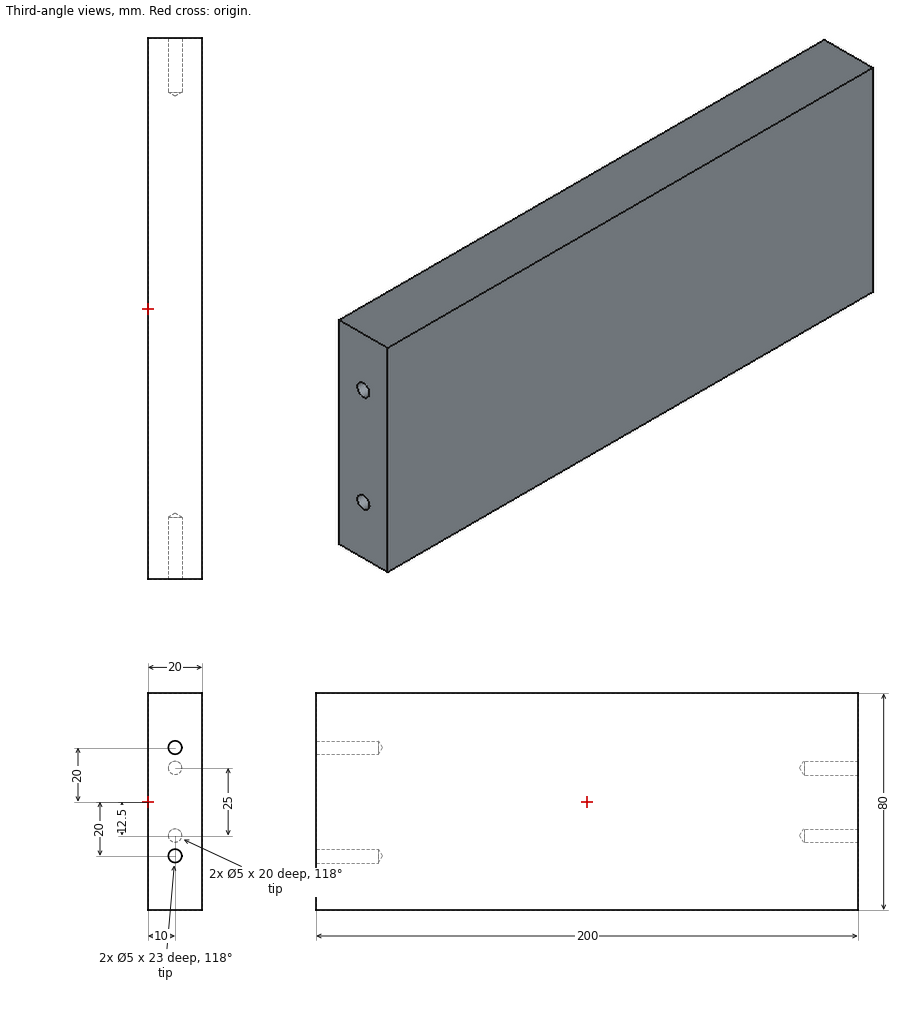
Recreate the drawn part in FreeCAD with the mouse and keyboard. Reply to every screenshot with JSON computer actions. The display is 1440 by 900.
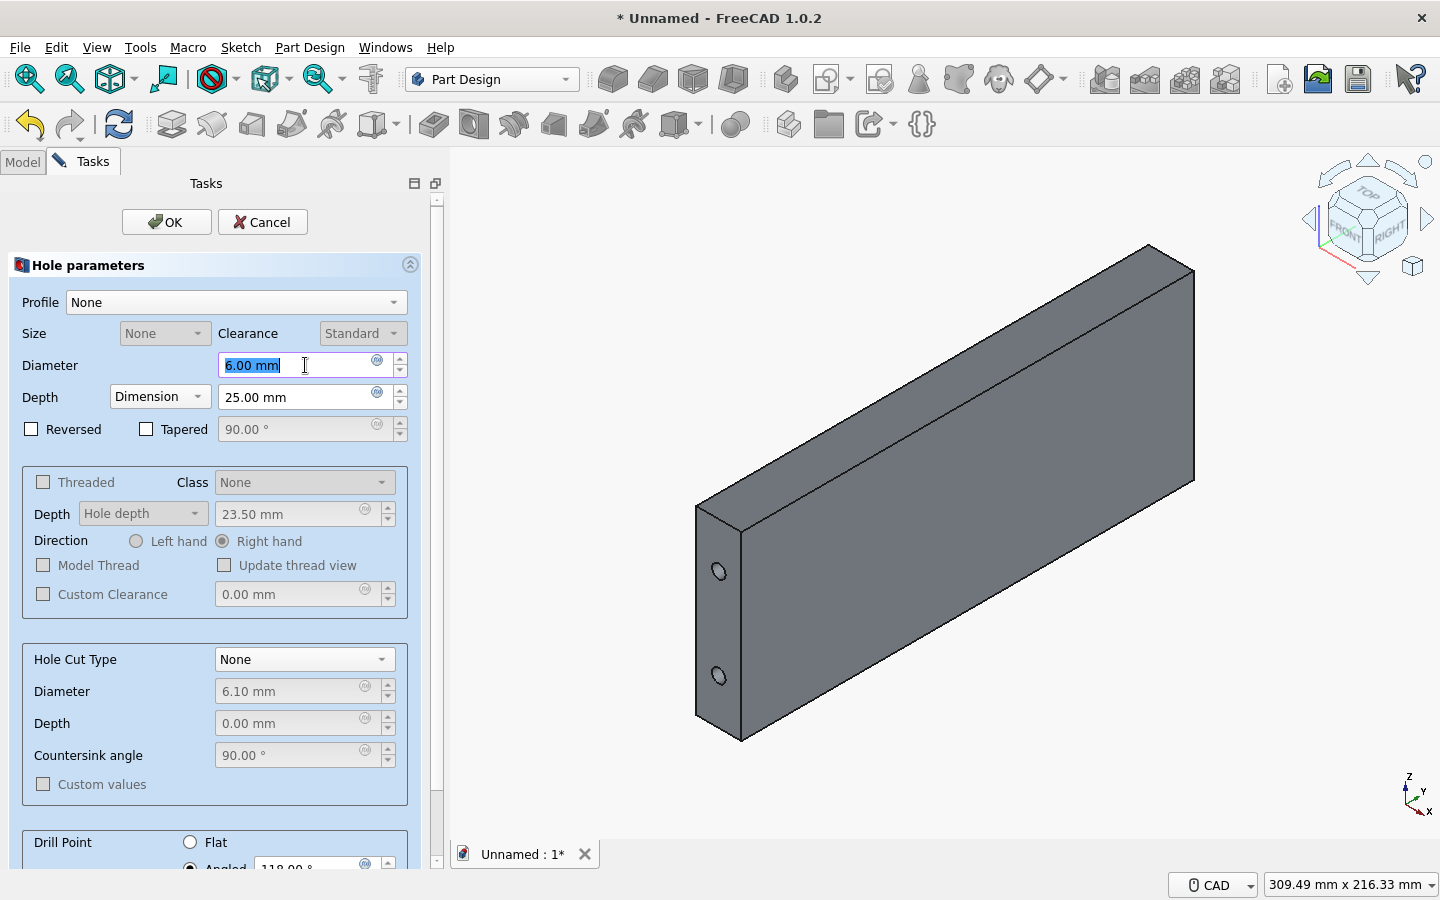
{"action": "type", "text": "5"}
{"action": "key", "text": "Tab"}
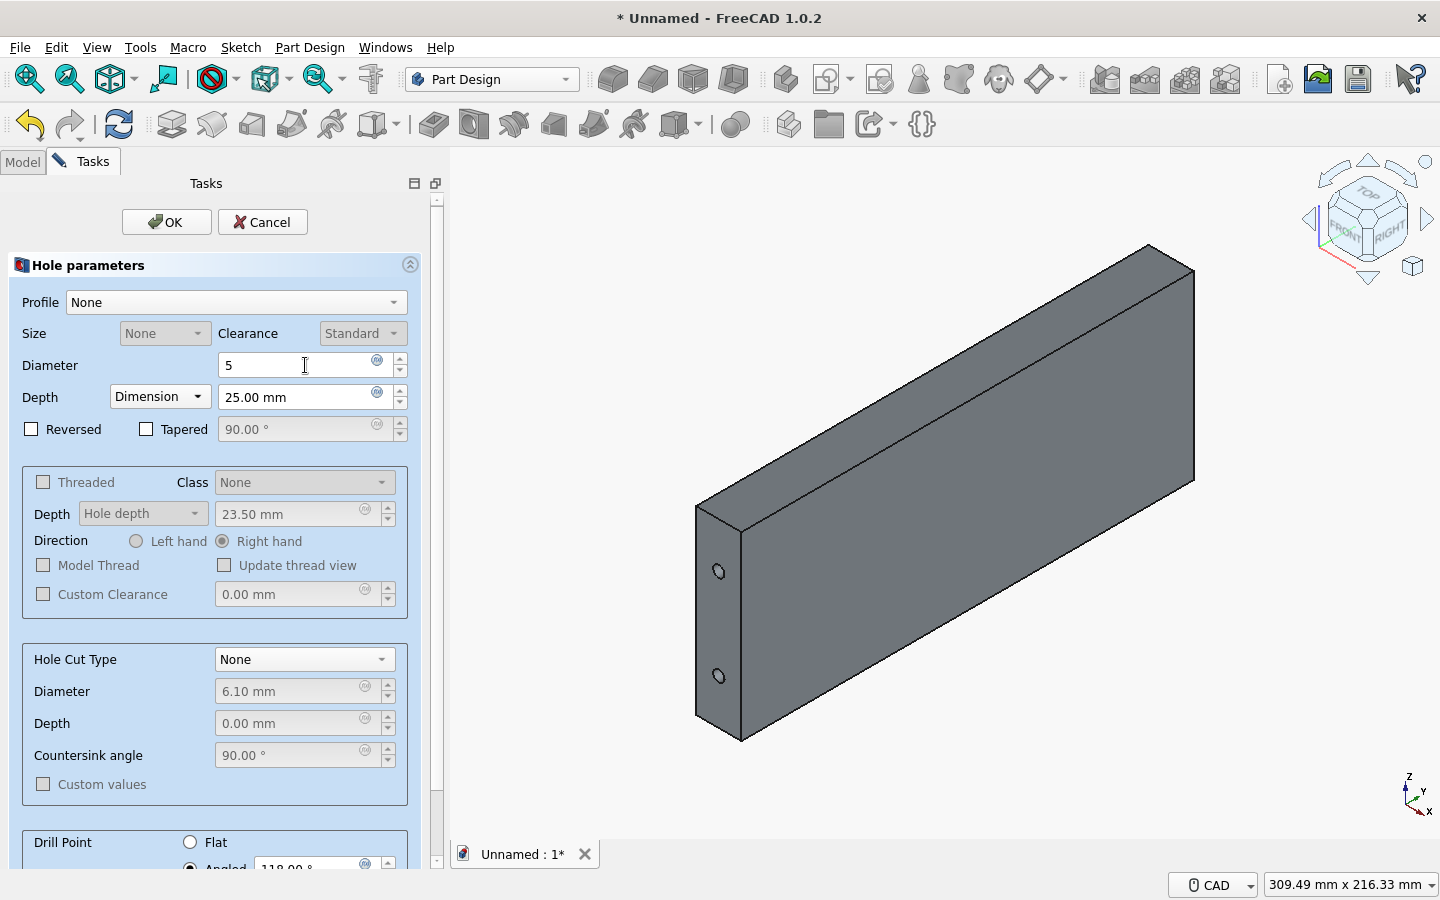
{"action": "triple_click", "coordinate": [305, 397]}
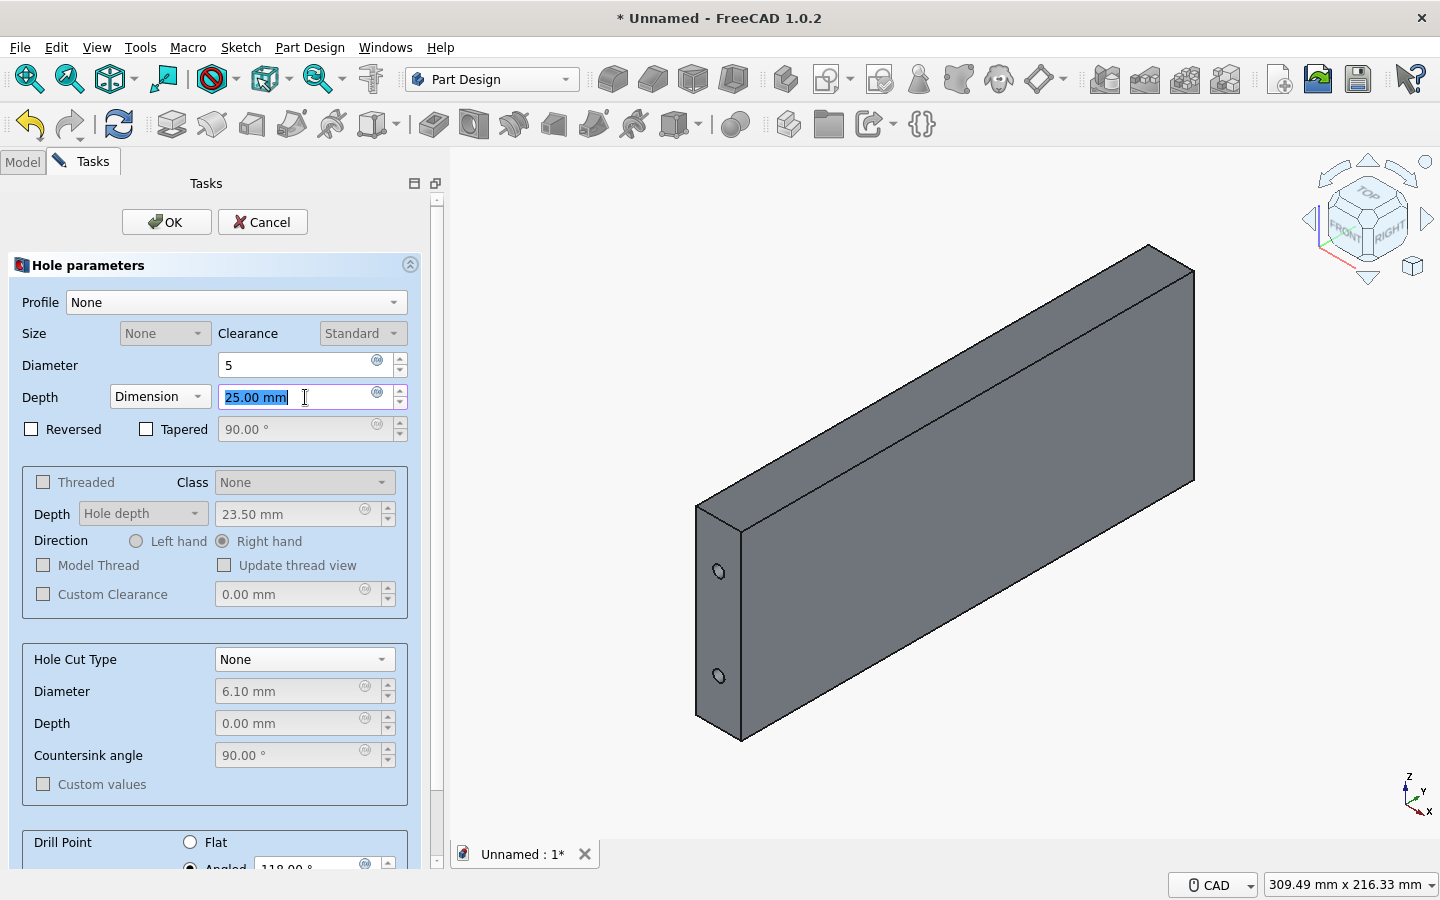
{"action": "type", "text": "23"}
{"action": "key", "text": "Tab"}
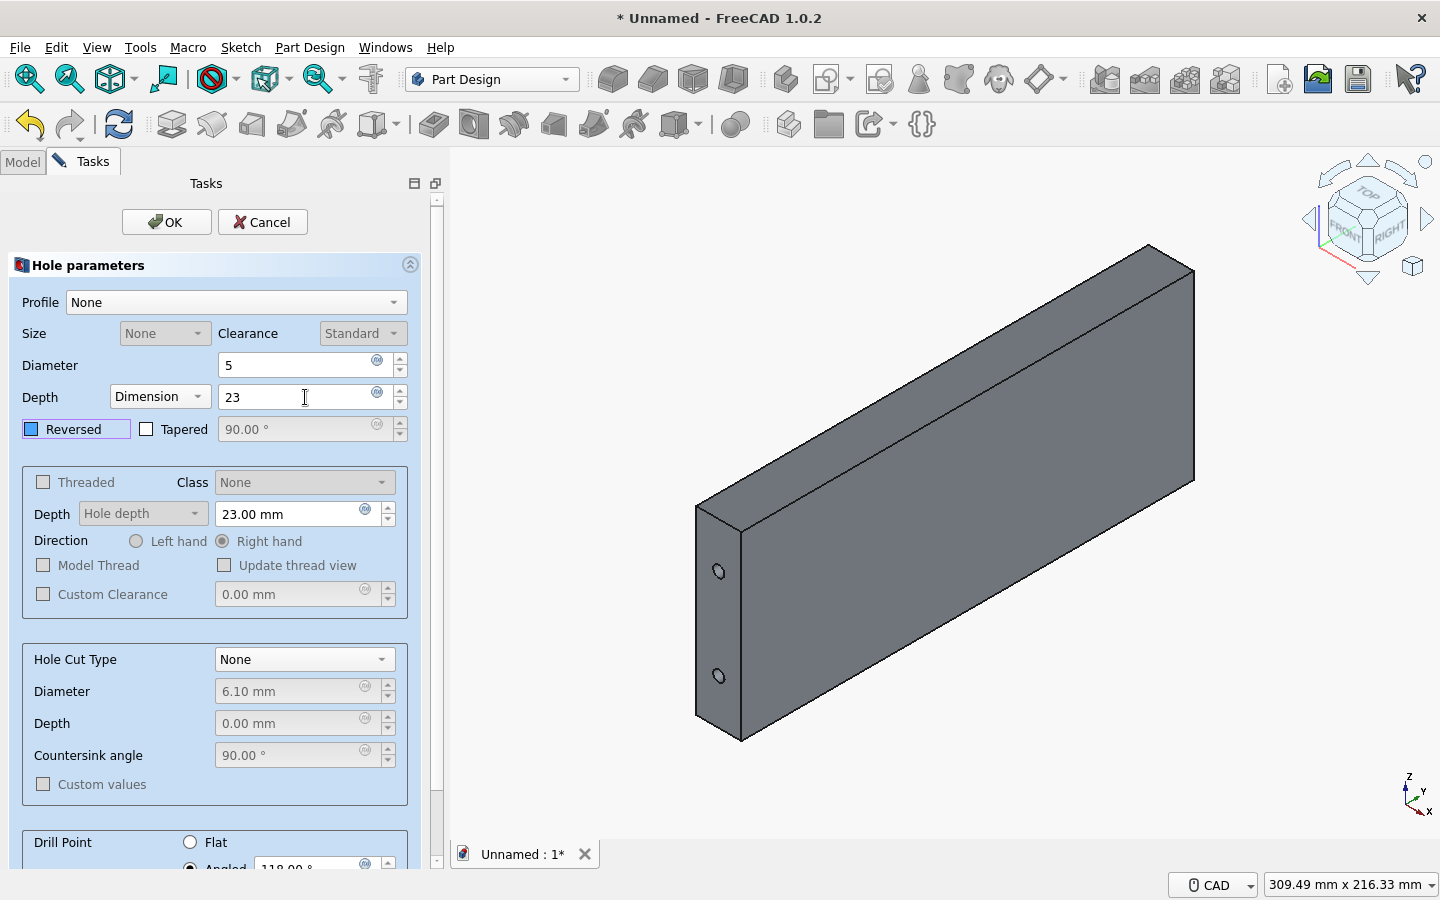
{"action": "left_click", "coordinate": [167, 222]}